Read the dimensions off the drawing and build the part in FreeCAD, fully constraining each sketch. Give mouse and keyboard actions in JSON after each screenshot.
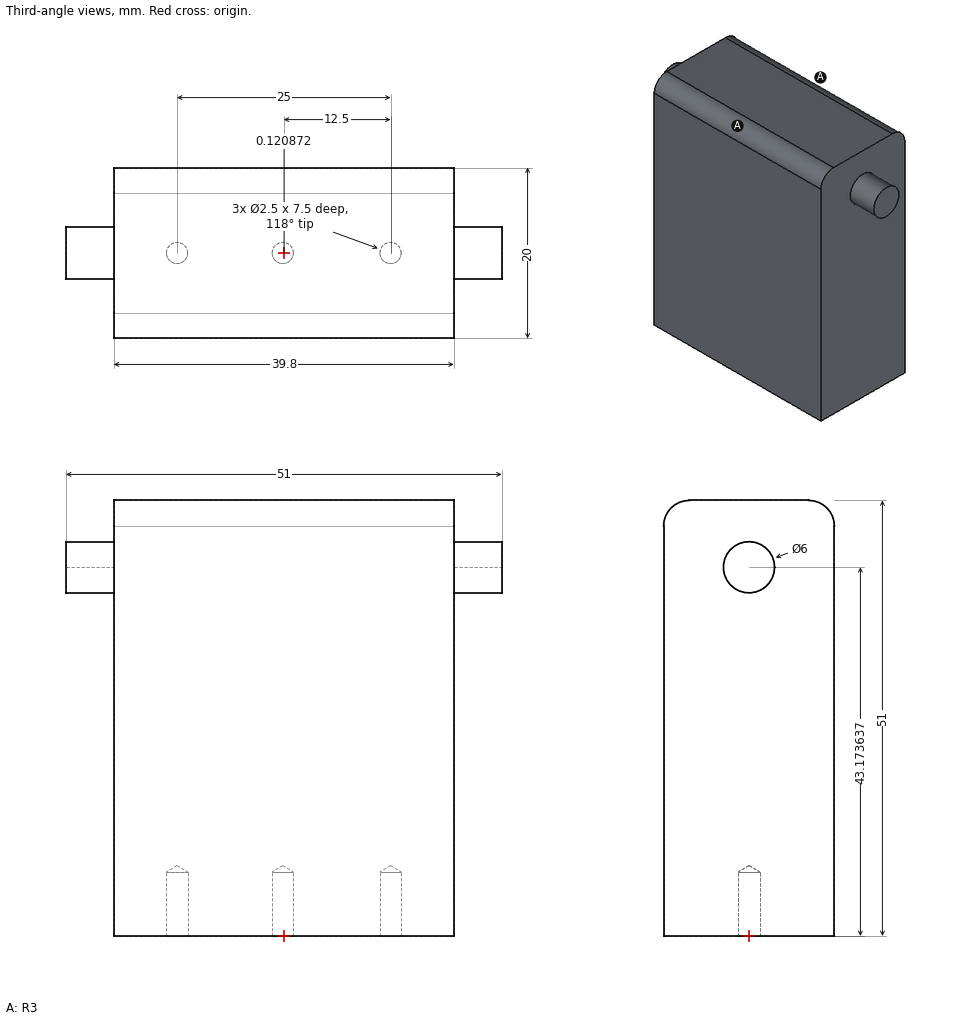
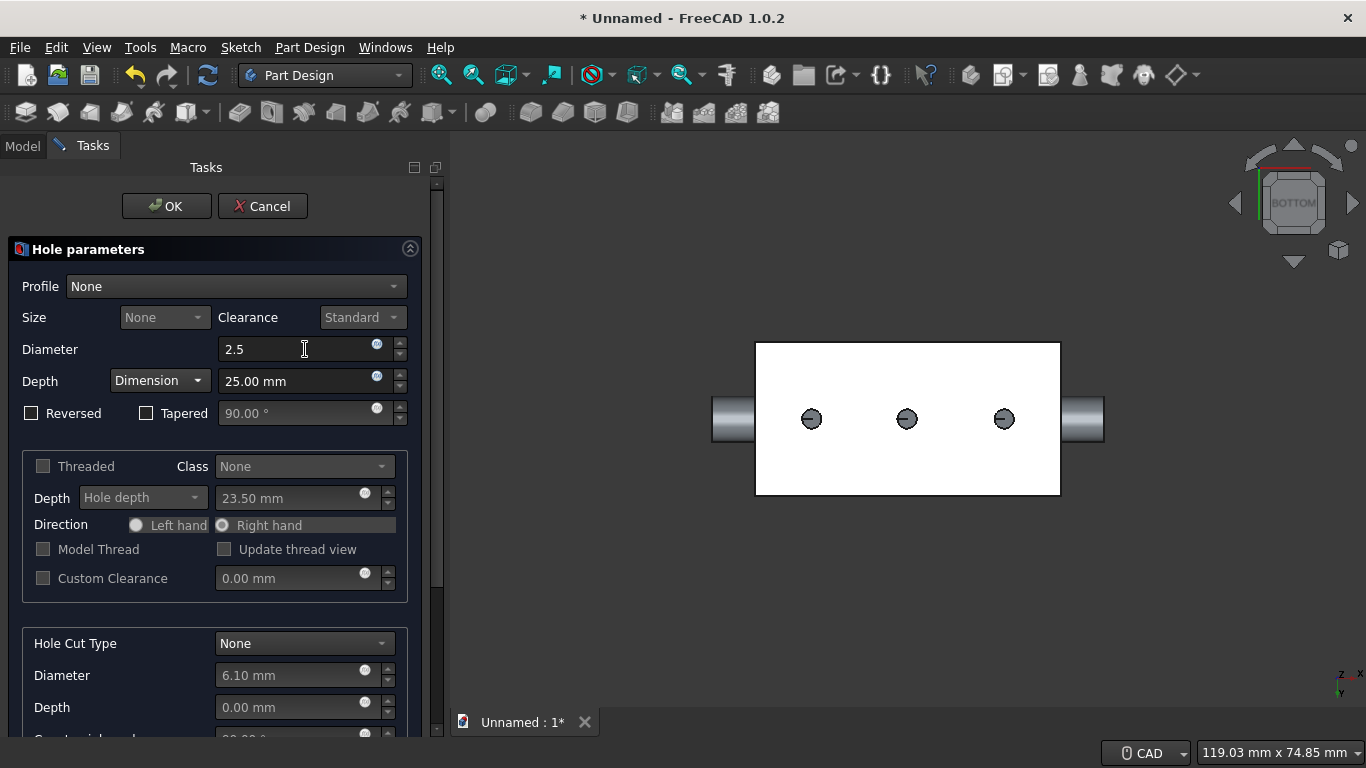
{"action": "triple_click", "coordinate": [305, 381]}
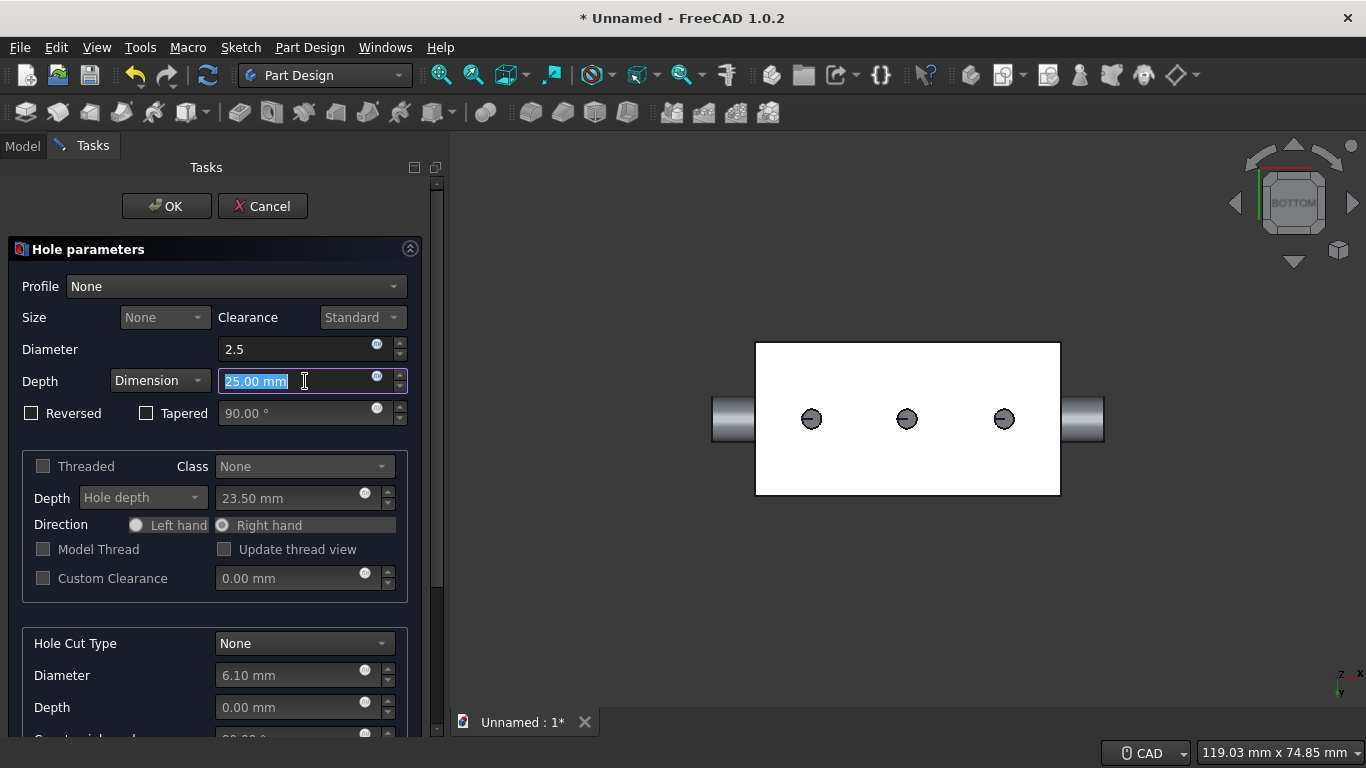
{"action": "type", "text": "7.5"}
{"action": "key", "text": "Tab"}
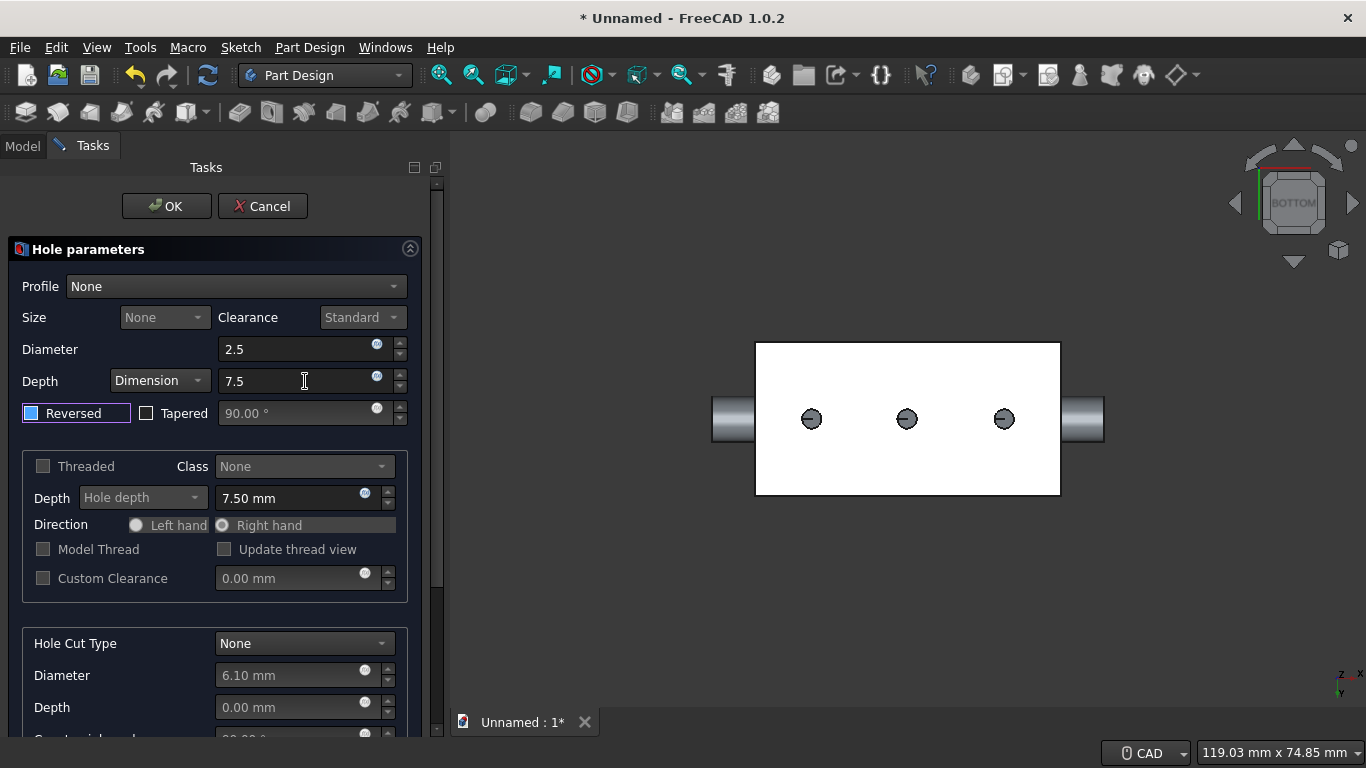
{"action": "left_click", "coordinate": [167, 206]}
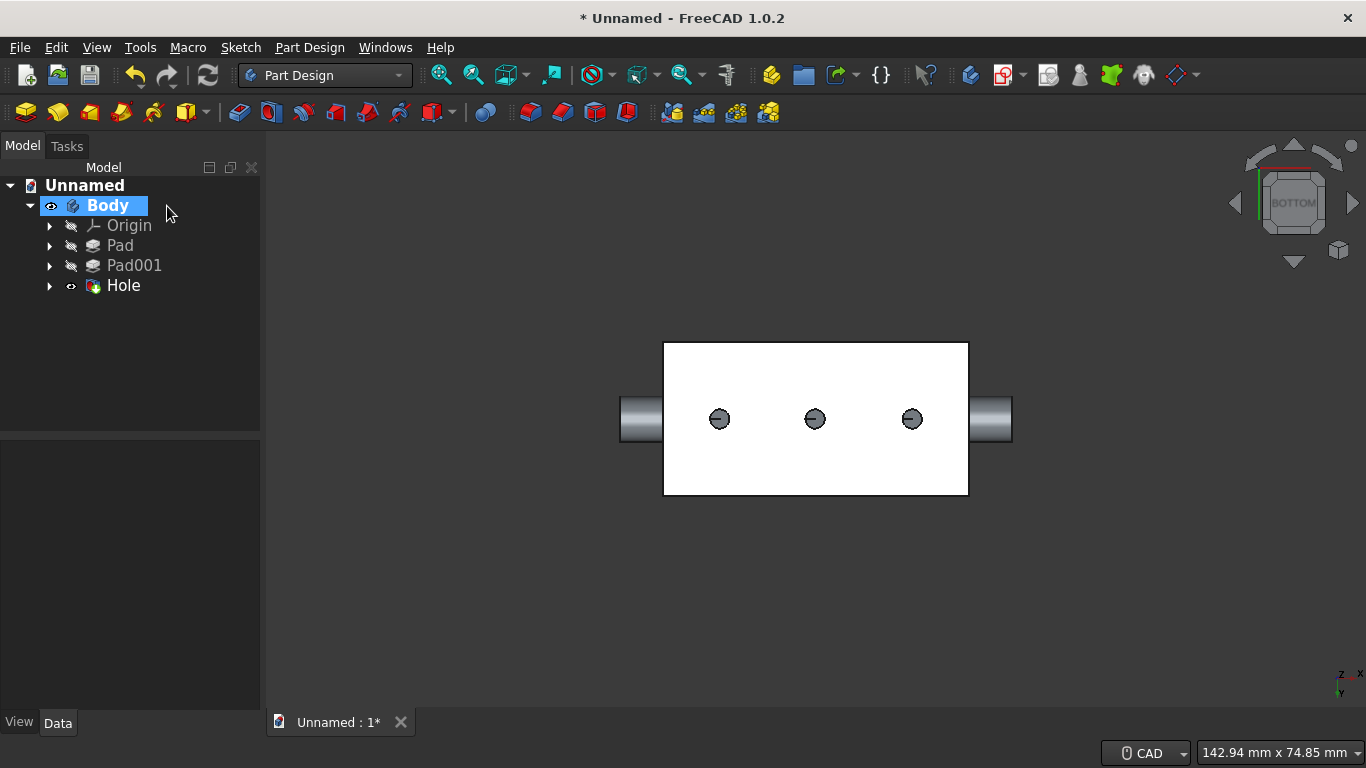
{"action": "key", "text": "v f"}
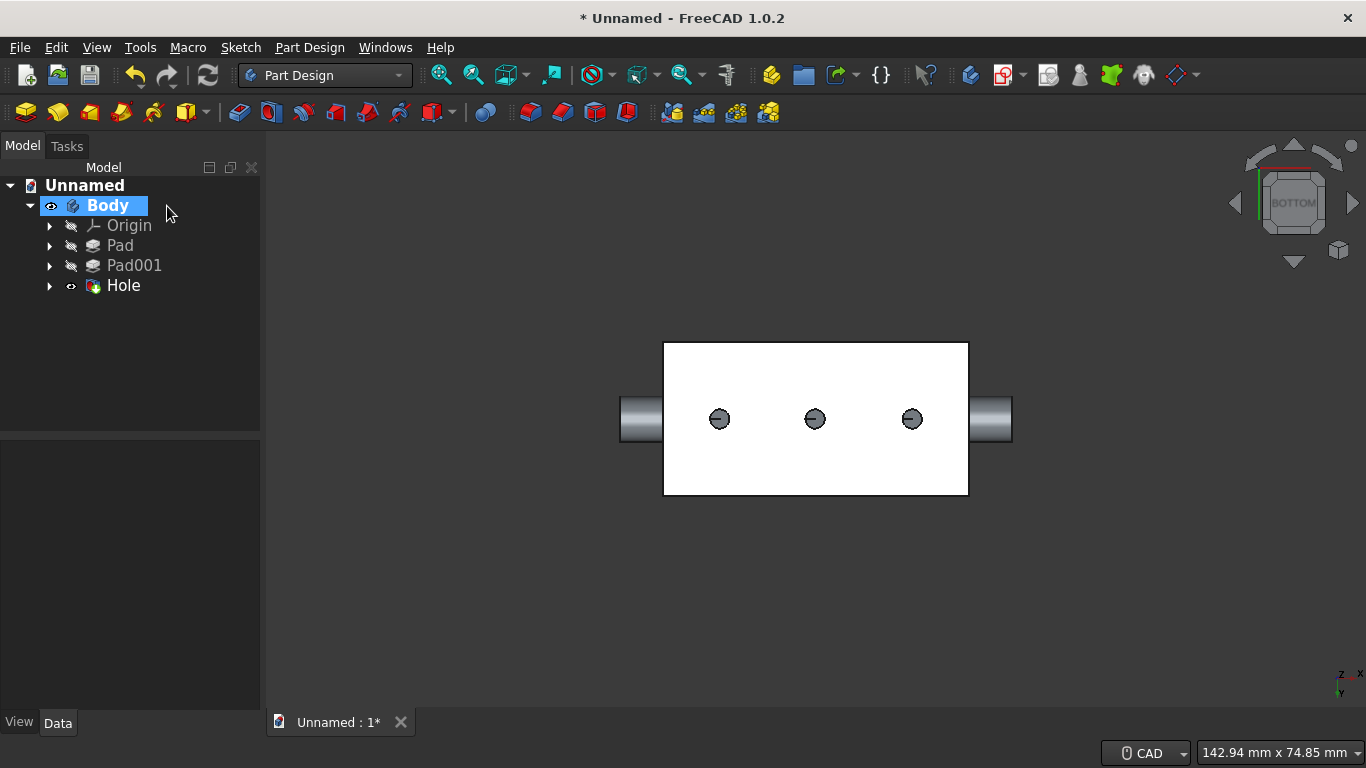
{"action": "key", "text": "0"}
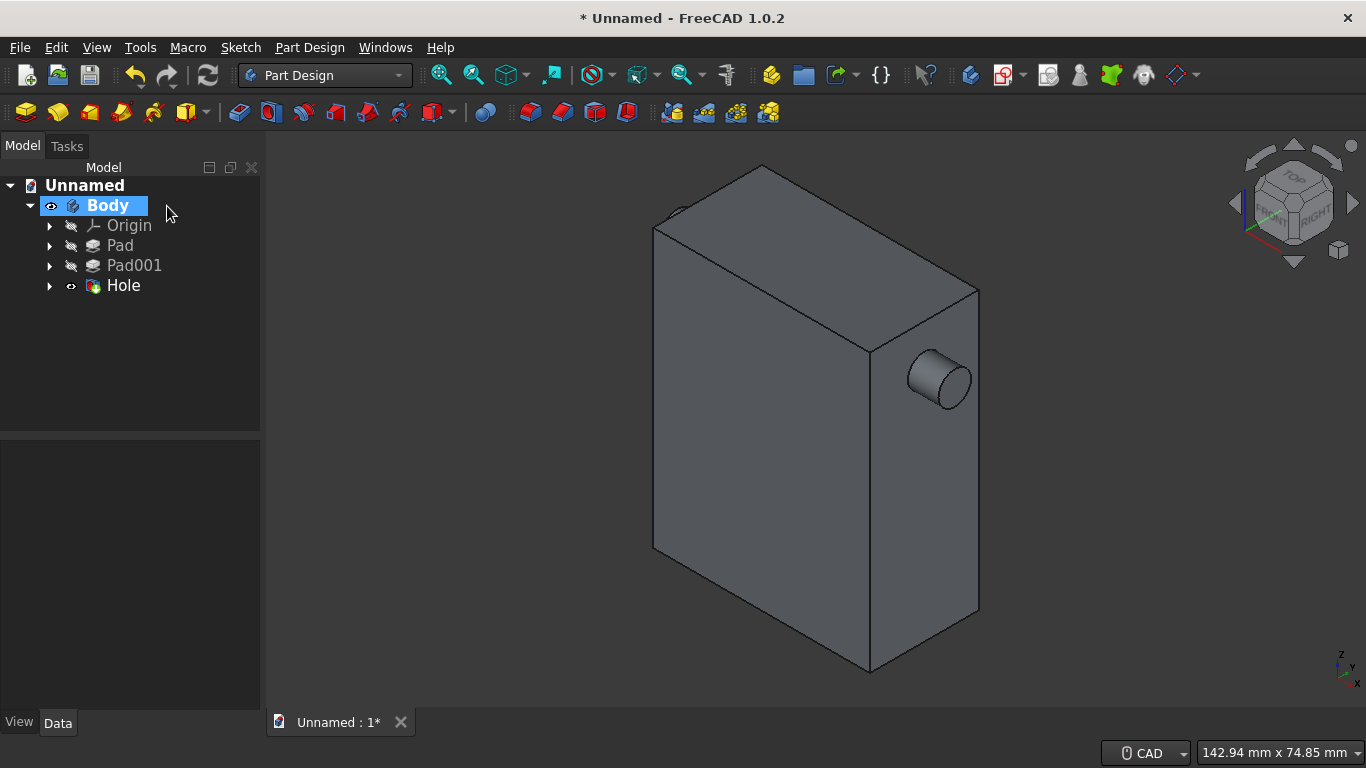
{"action": "left_click", "coordinate": [762, 289]}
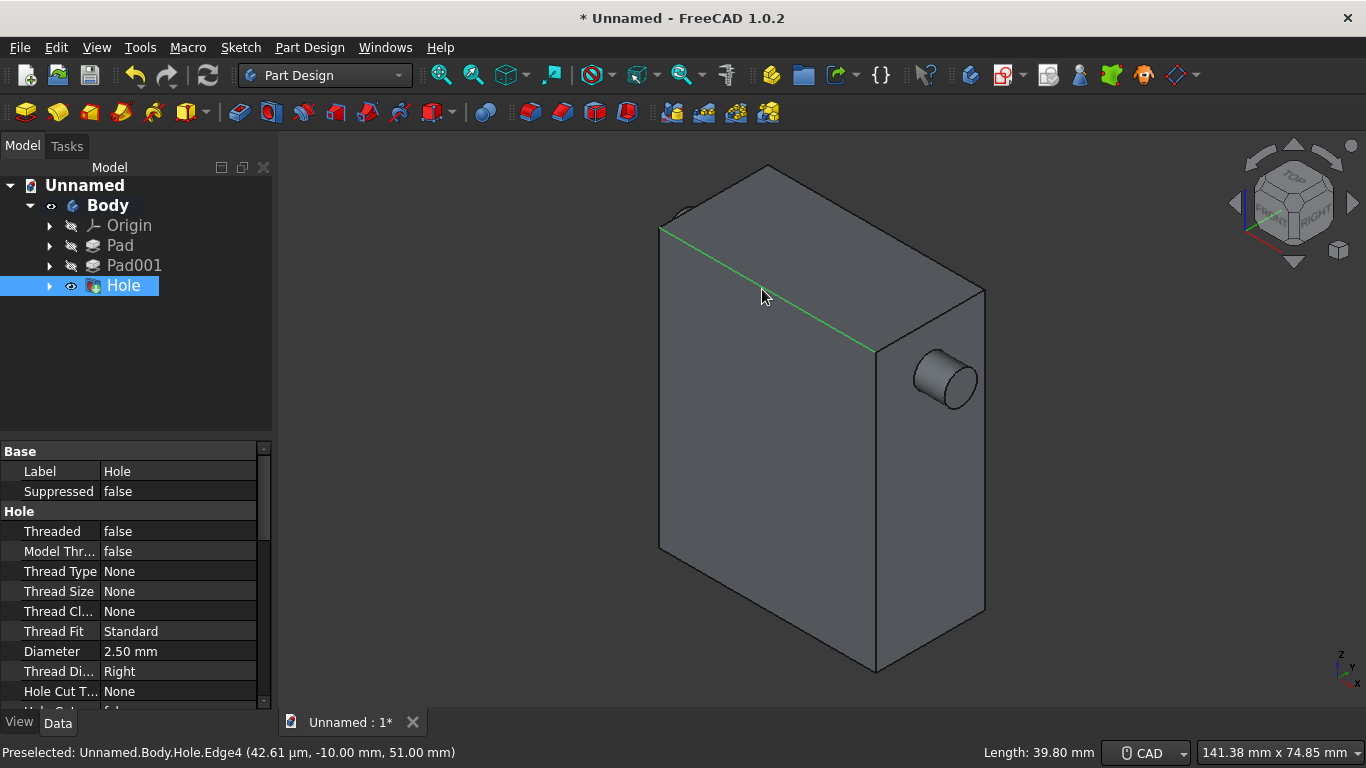
{"action": "key", "text": "2"}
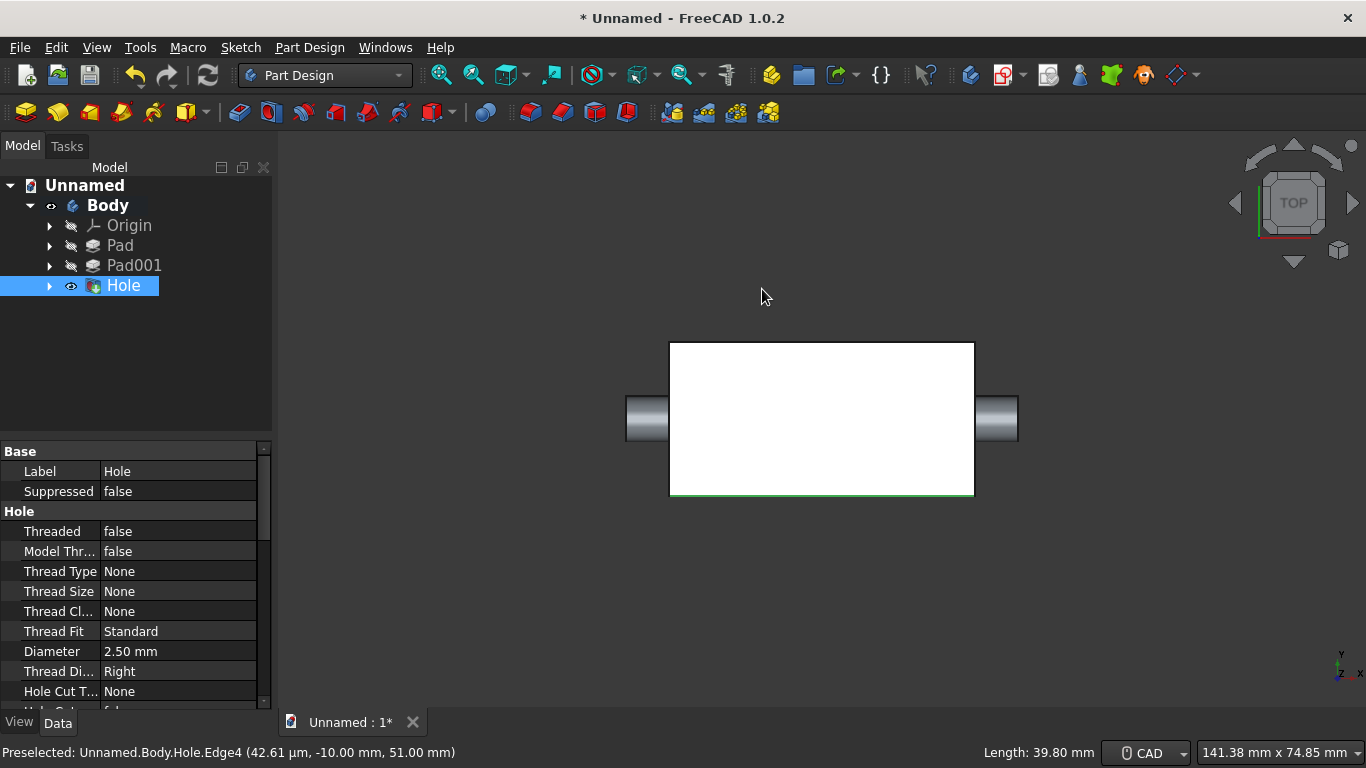
{"action": "key", "text": "v f"}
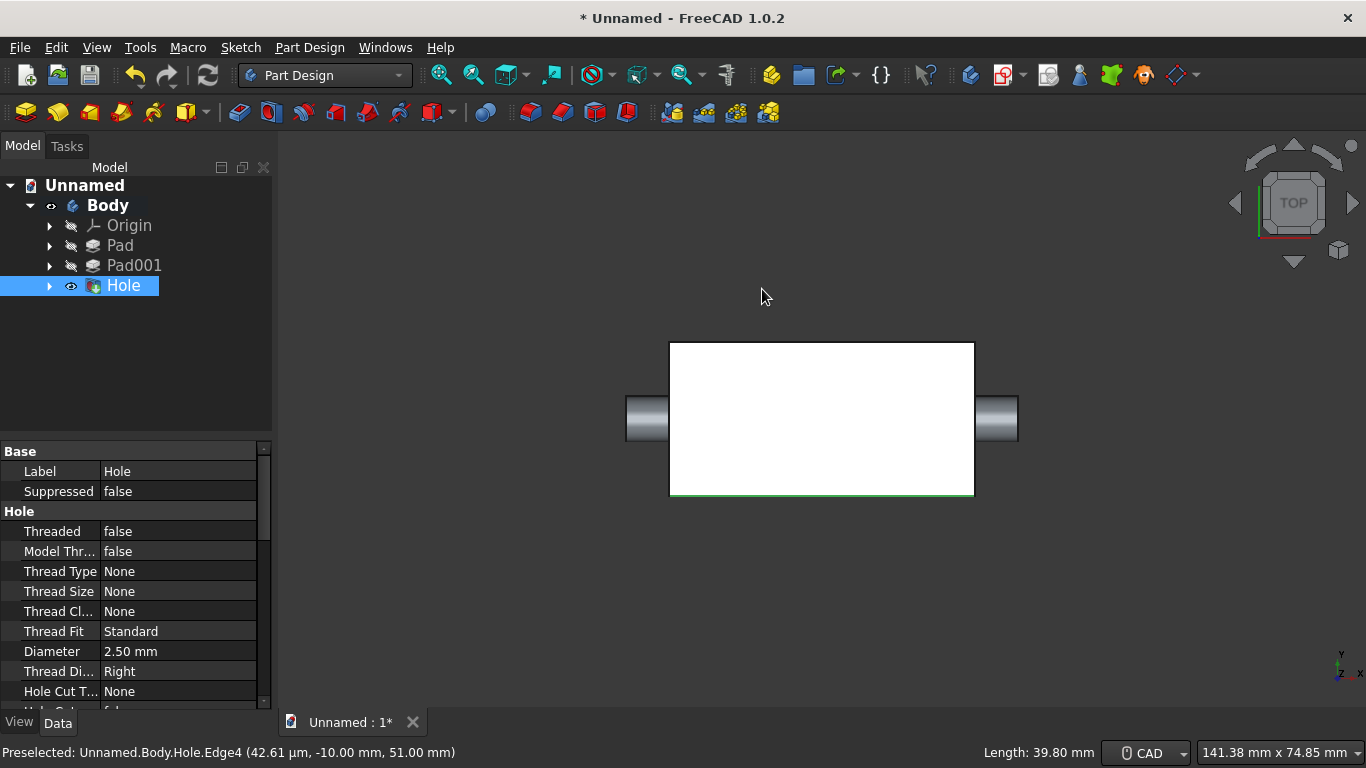
{"action": "left_click", "coordinate": [822, 341], "text": "ctrl"}